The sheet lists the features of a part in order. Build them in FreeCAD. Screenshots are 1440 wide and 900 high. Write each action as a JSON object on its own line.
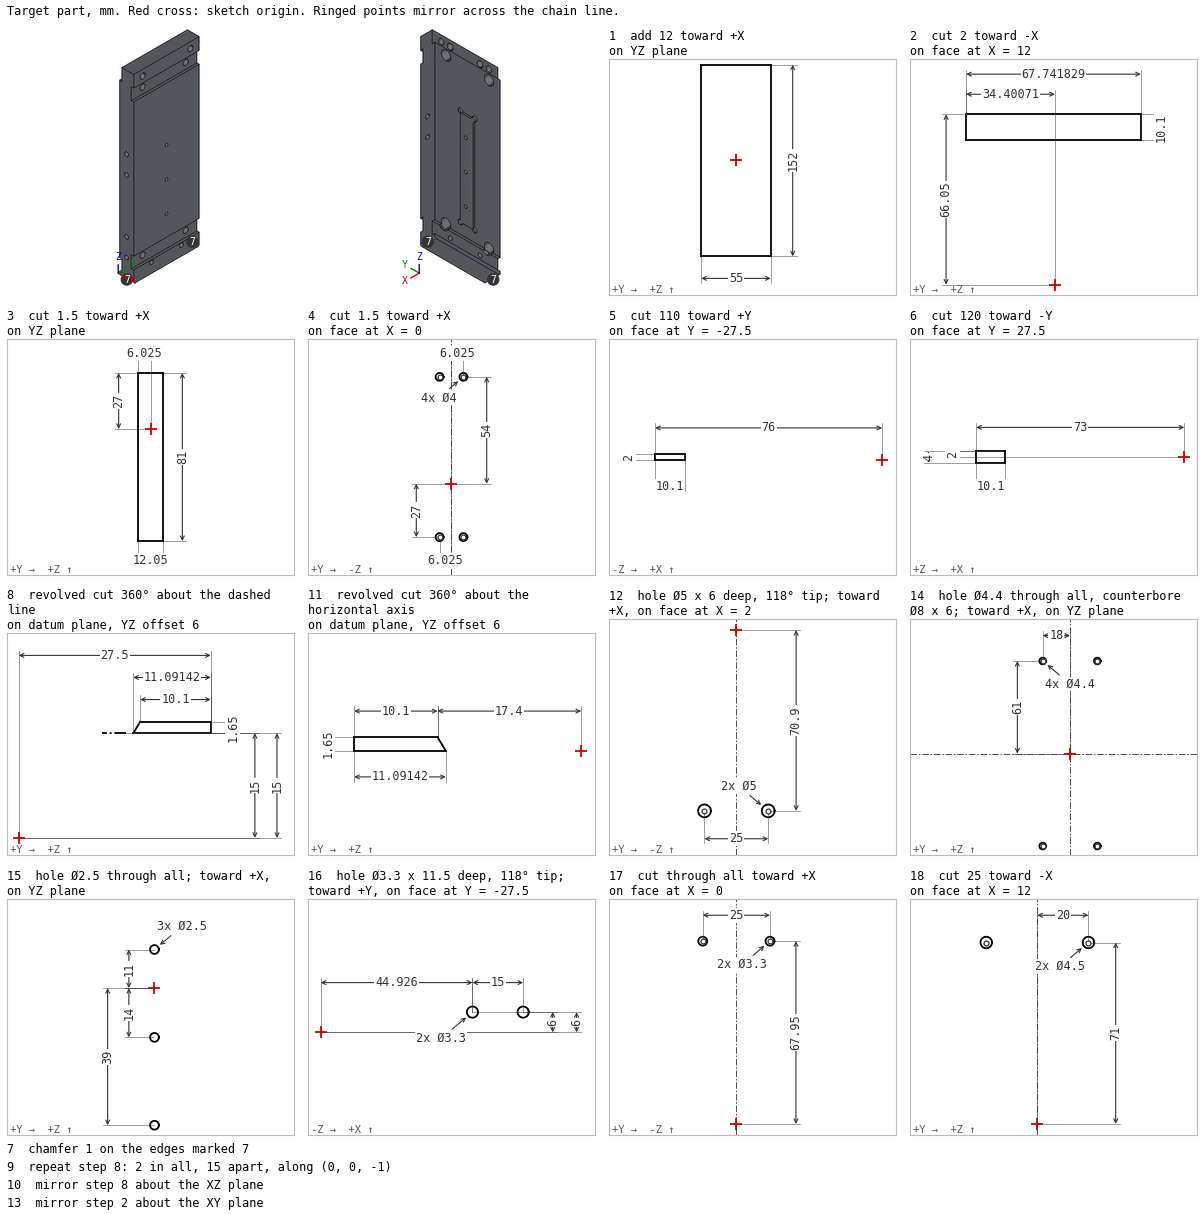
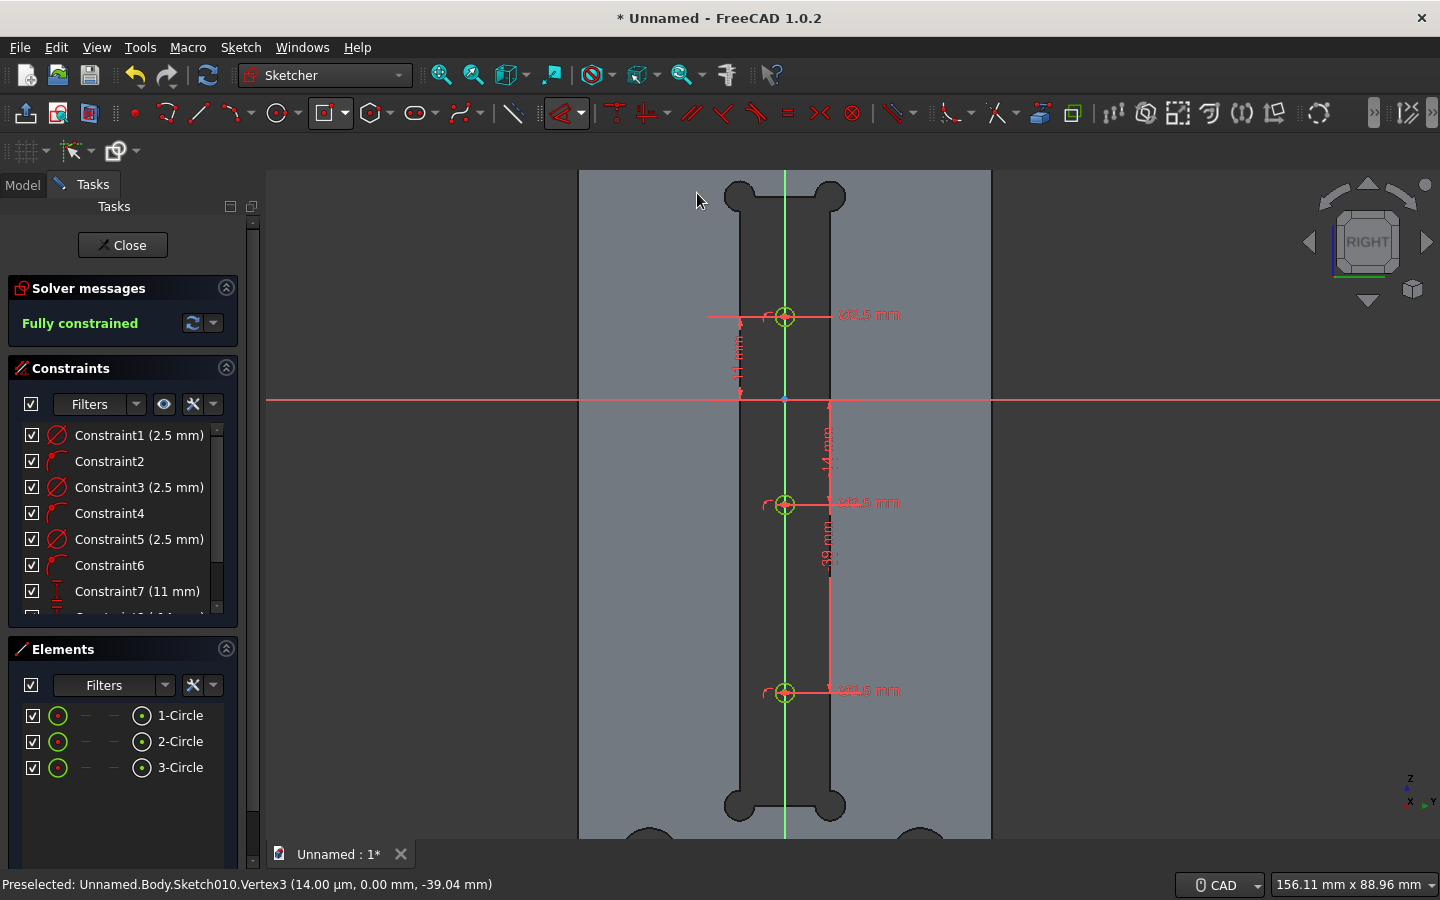
{"action": "left_click", "coordinate": [123, 245]}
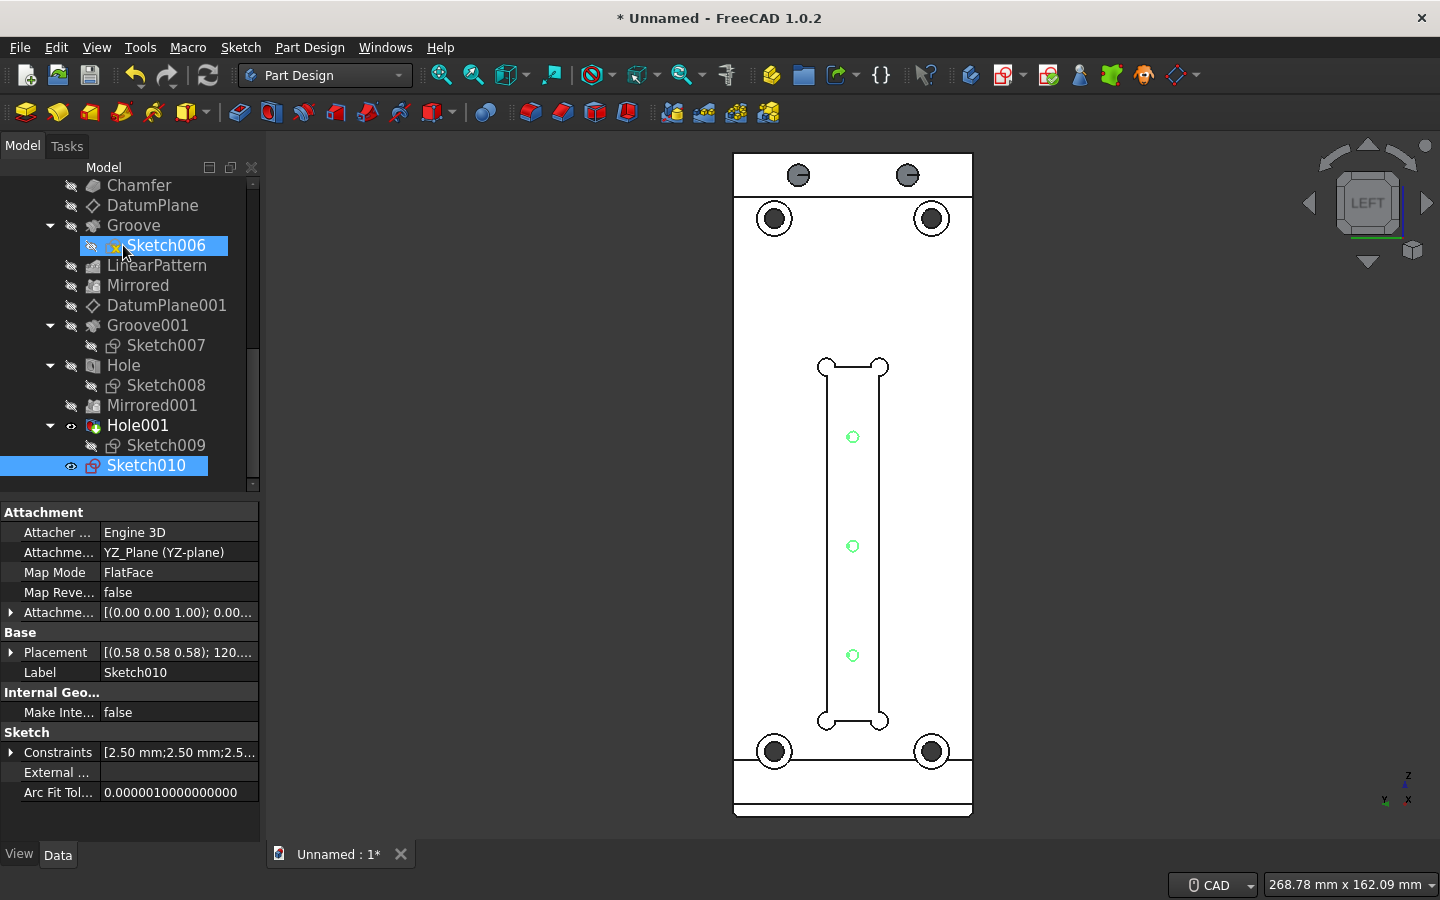
{"action": "left_click", "coordinate": [272, 112]}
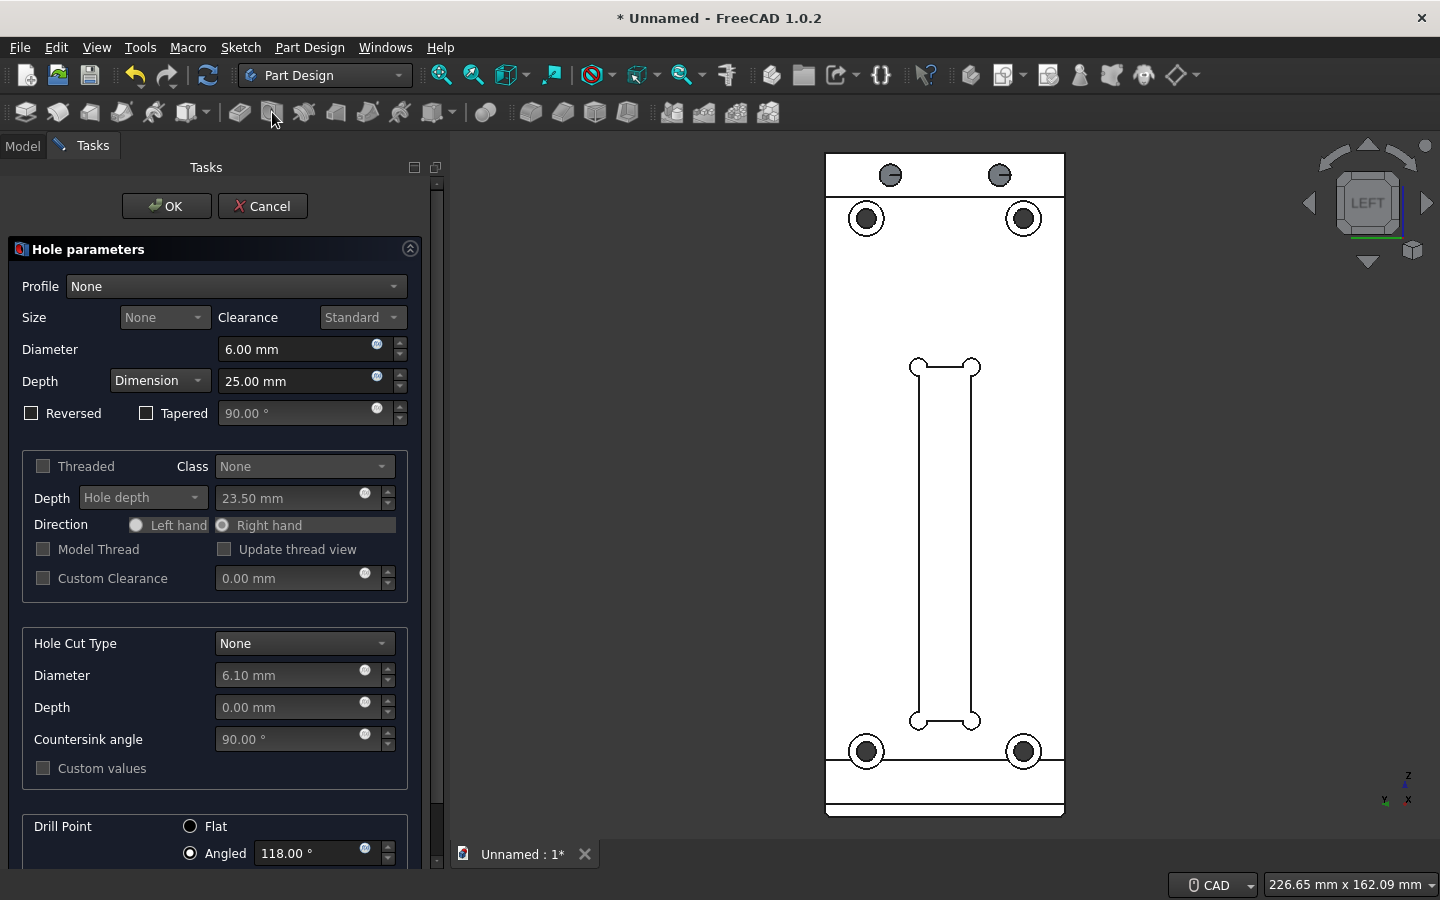
{"action": "triple_click", "coordinate": [305, 349]}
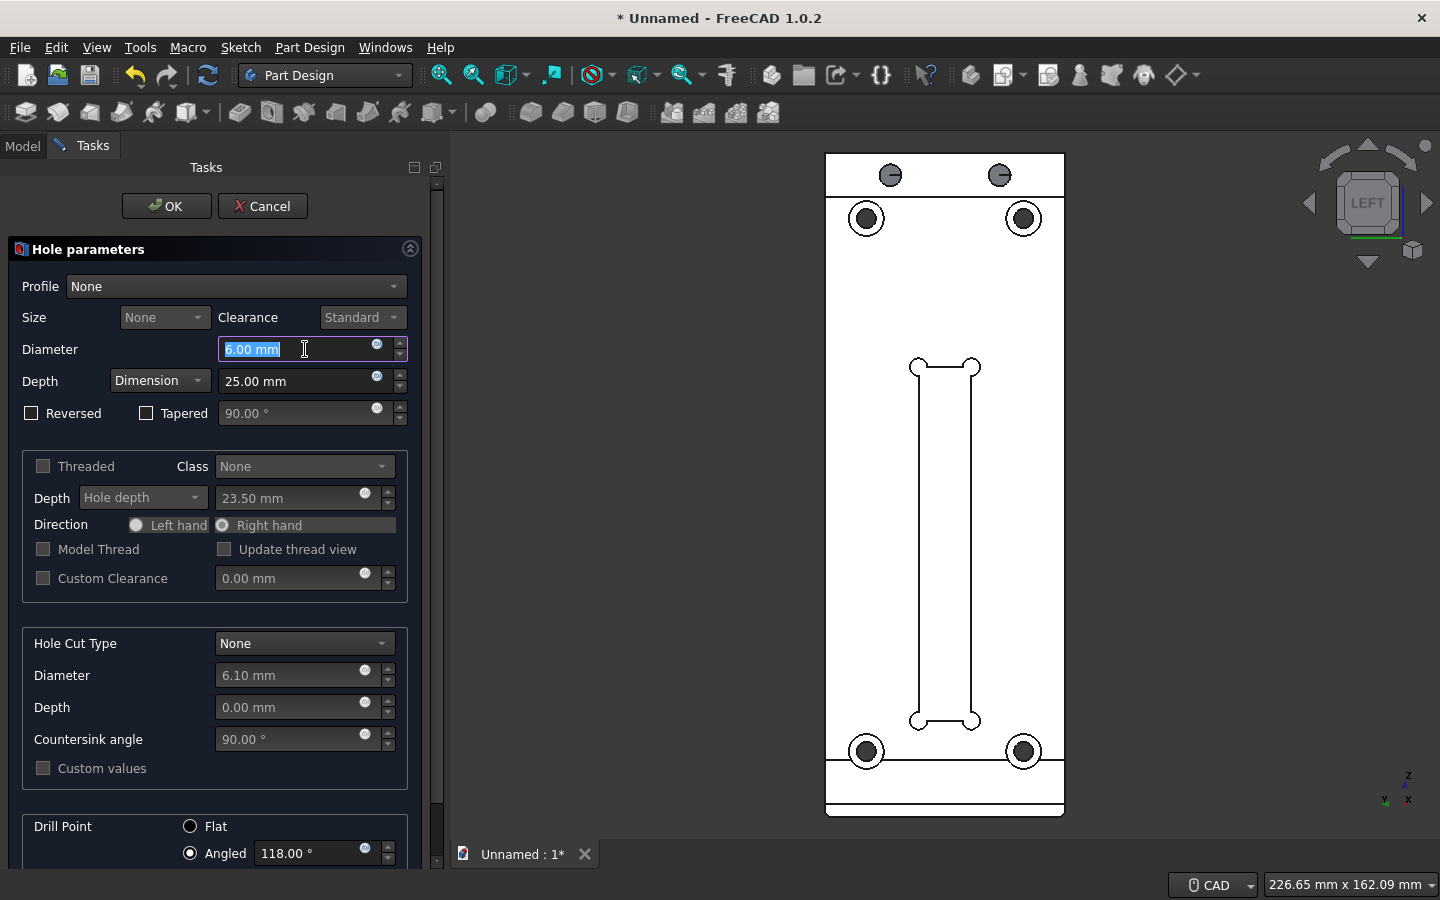
{"action": "type", "text": "2.5"}
{"action": "key", "text": "Tab"}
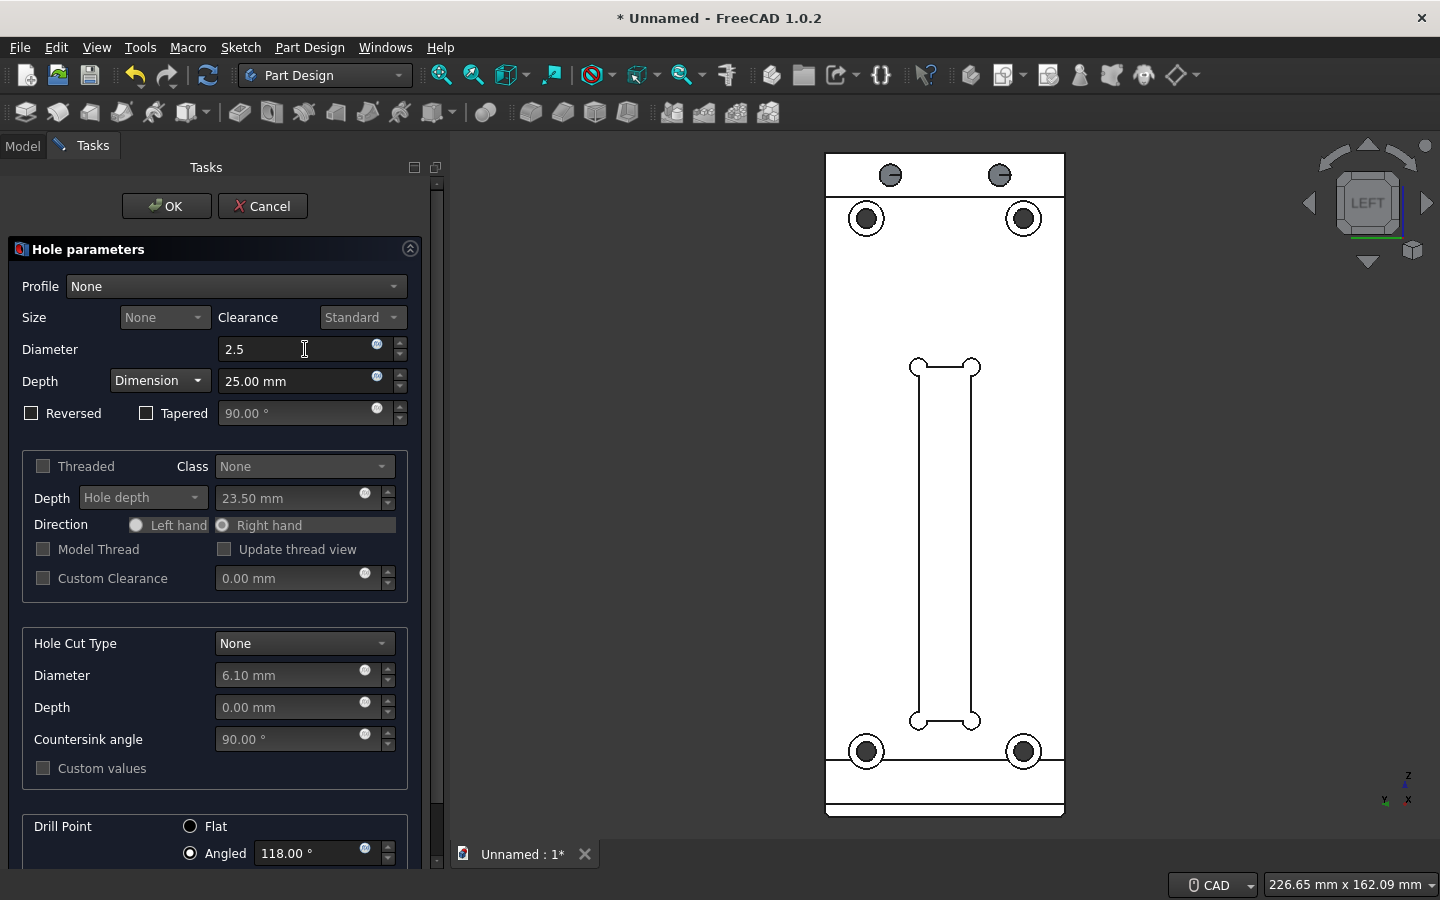
{"action": "left_click", "coordinate": [161, 380]}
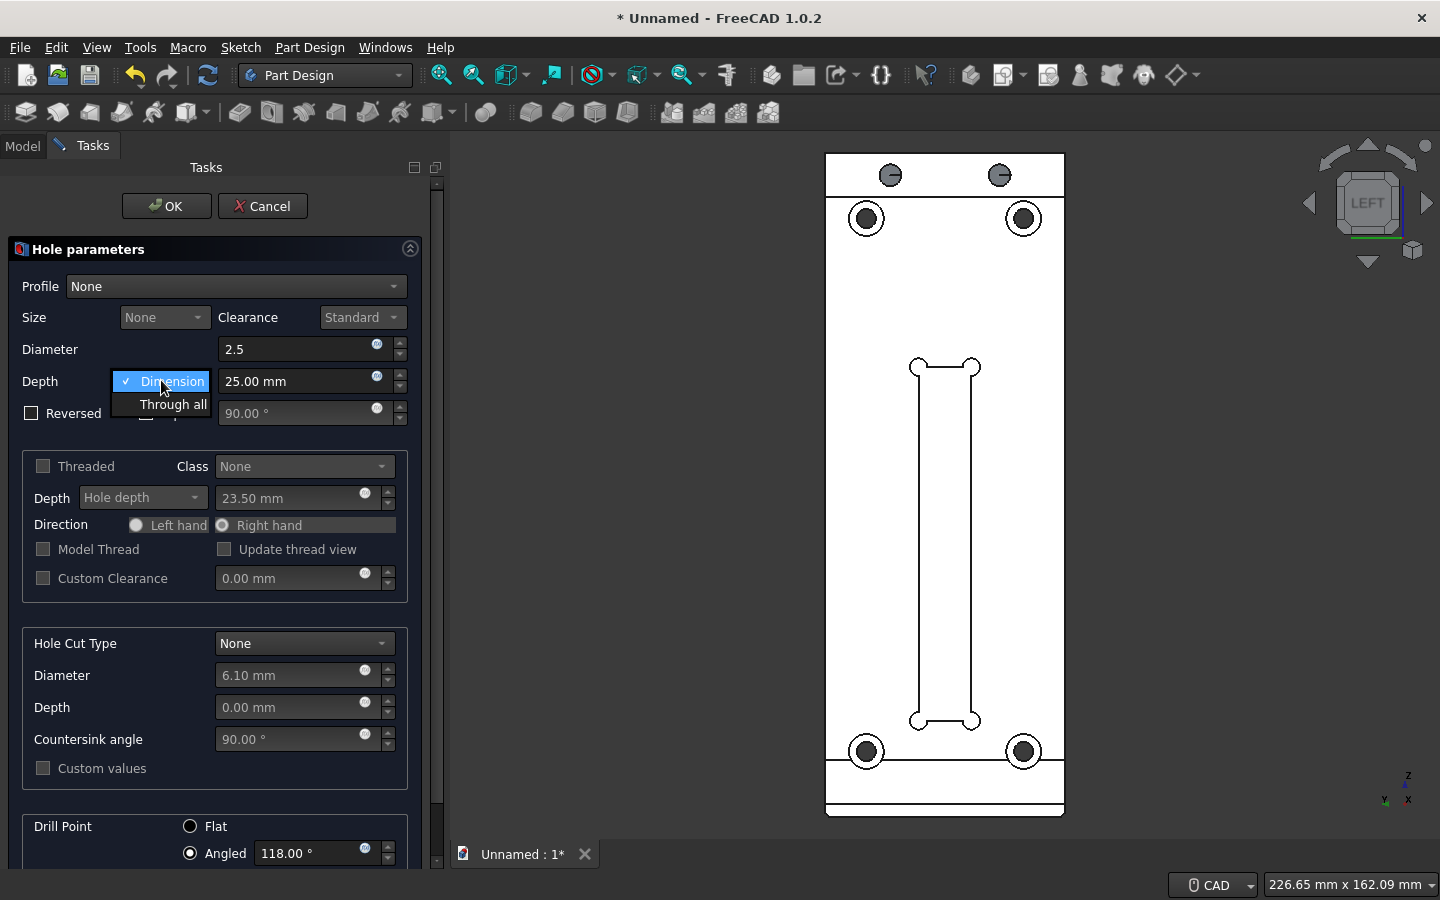
{"action": "left_click", "coordinate": [160, 404]}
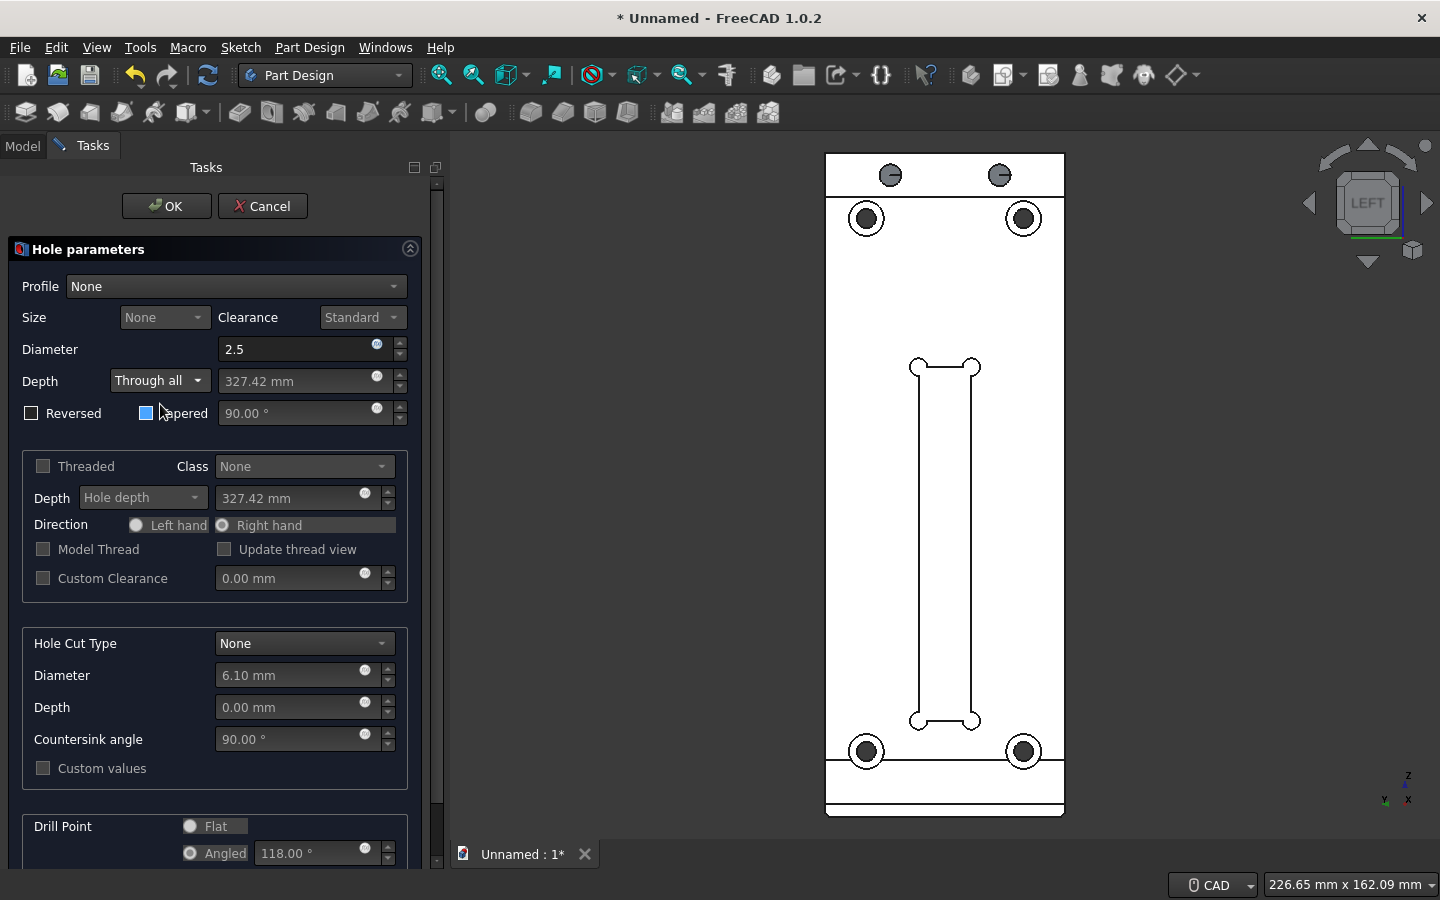
{"action": "left_click", "coordinate": [30, 413]}